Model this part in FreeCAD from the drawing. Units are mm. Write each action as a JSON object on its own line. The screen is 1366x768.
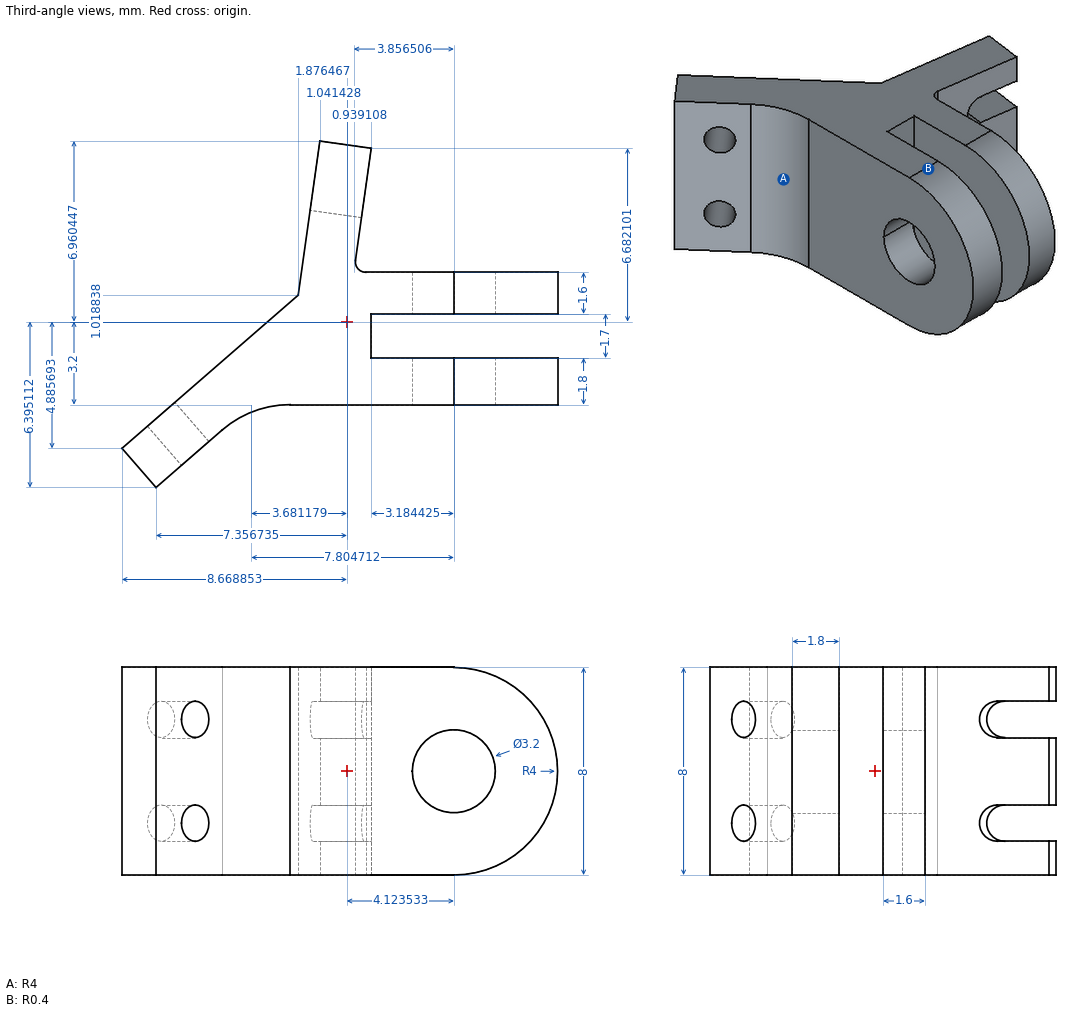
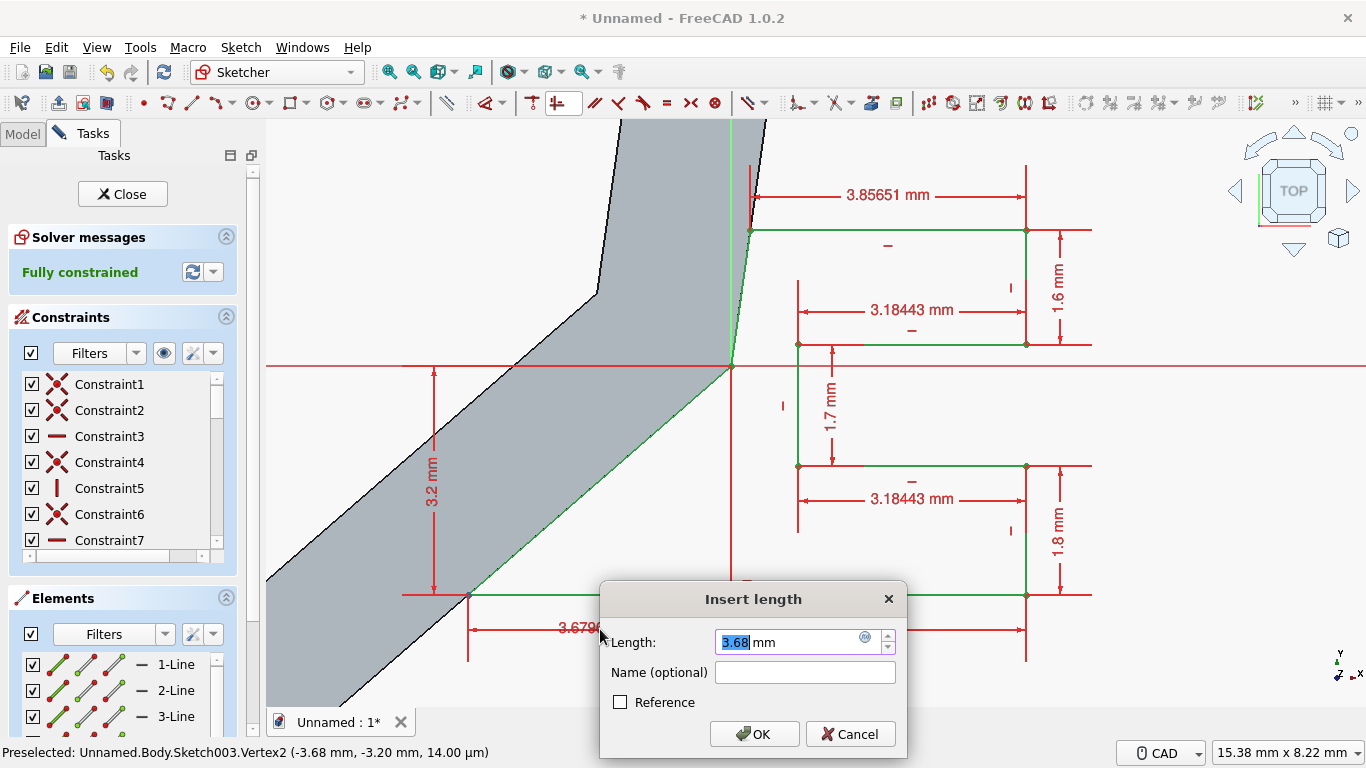
{"action": "type", "text": "3.681179"}
{"action": "key", "text": "Return"}
{"action": "key", "text": "Escape"}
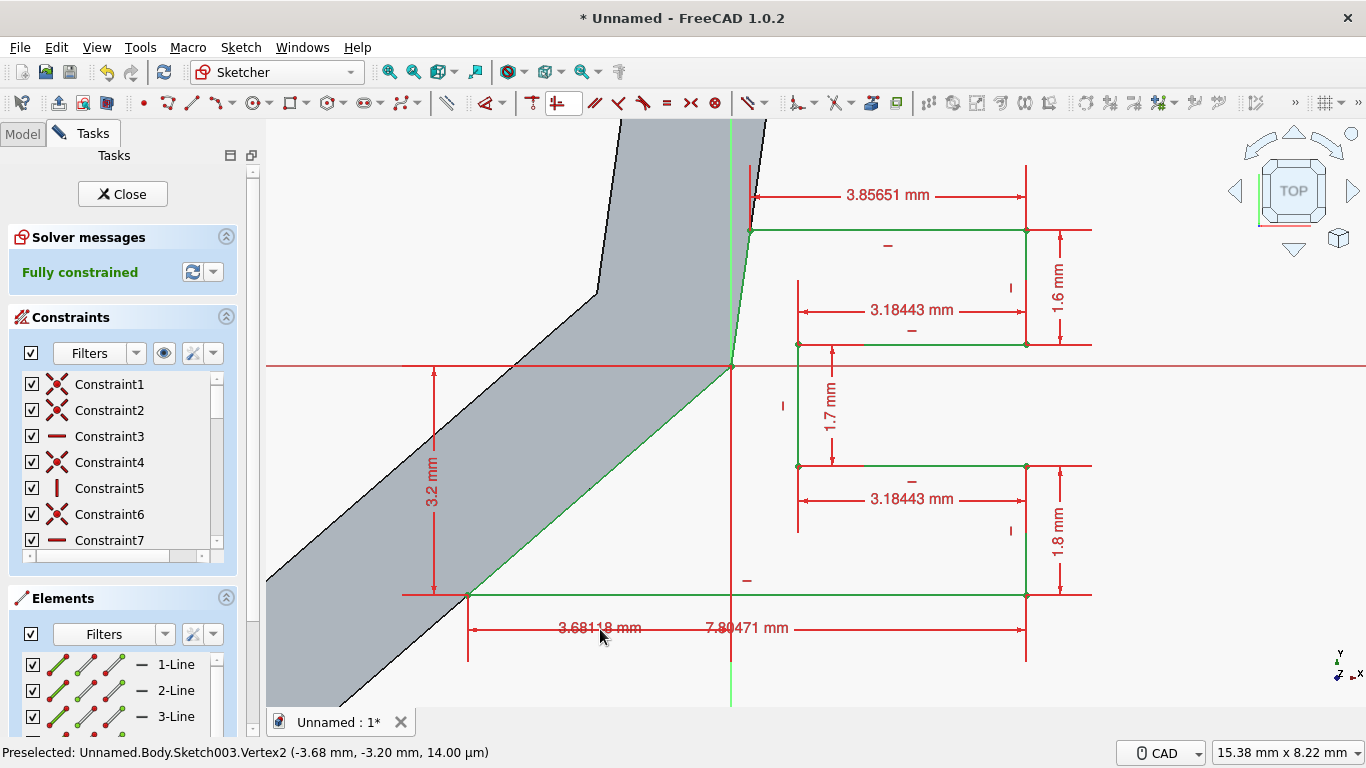
{"action": "left_click", "coordinate": [123, 194]}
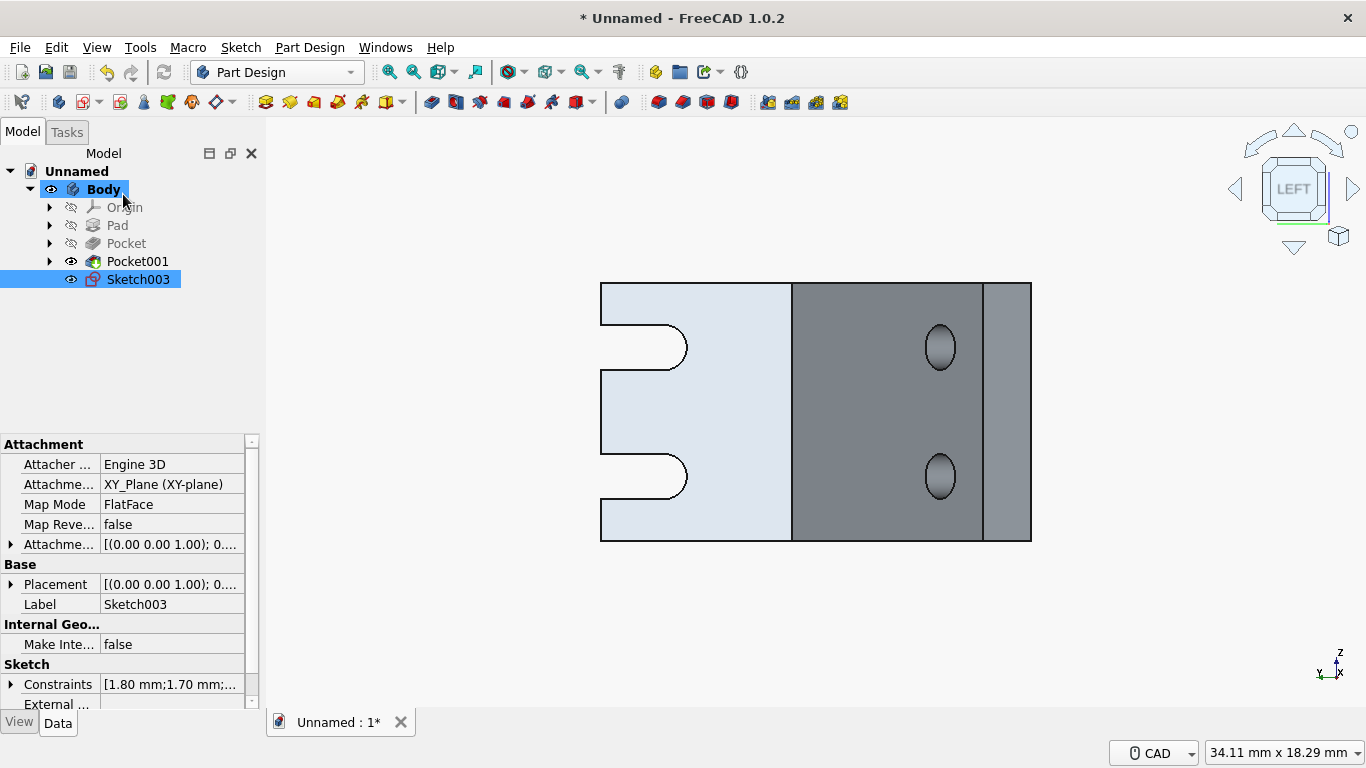
{"action": "left_click", "coordinate": [266, 102]}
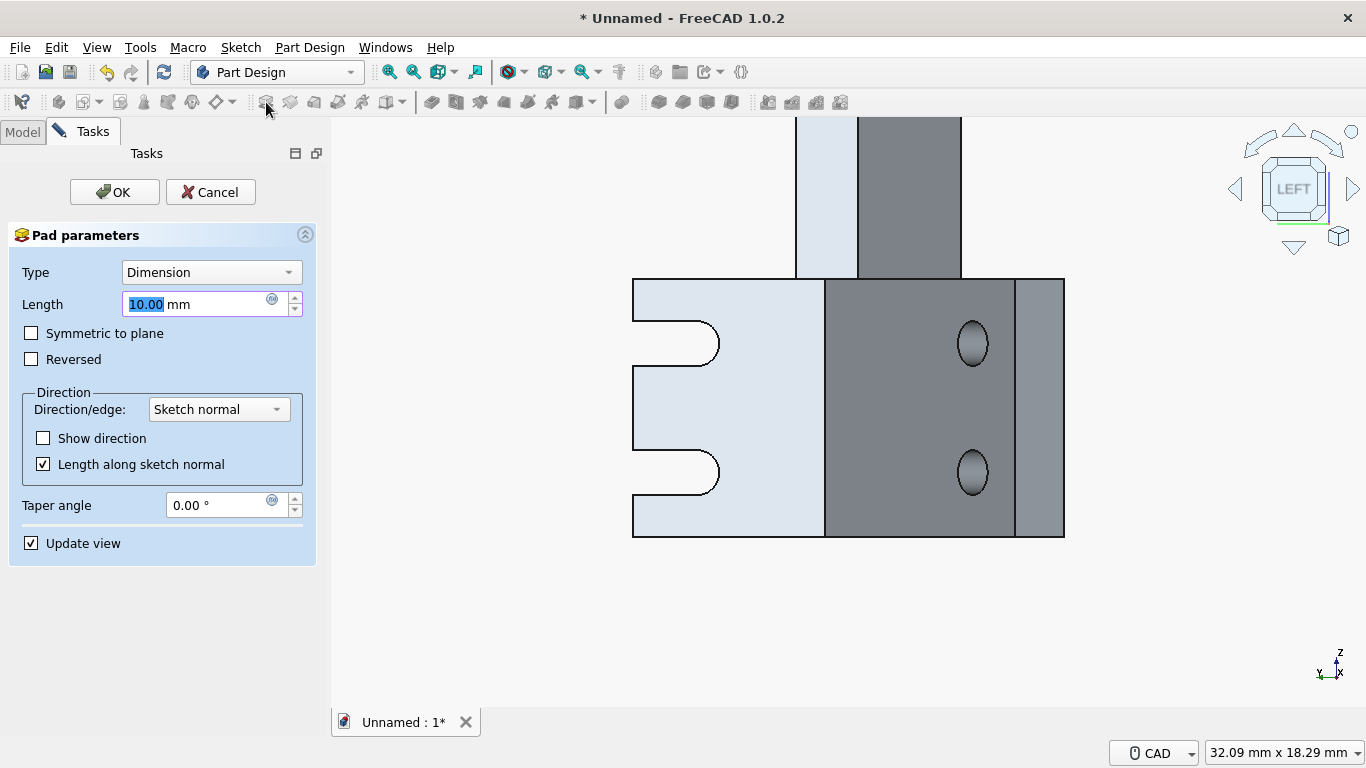
{"action": "type", "text": "8"}
{"action": "key", "text": "Tab"}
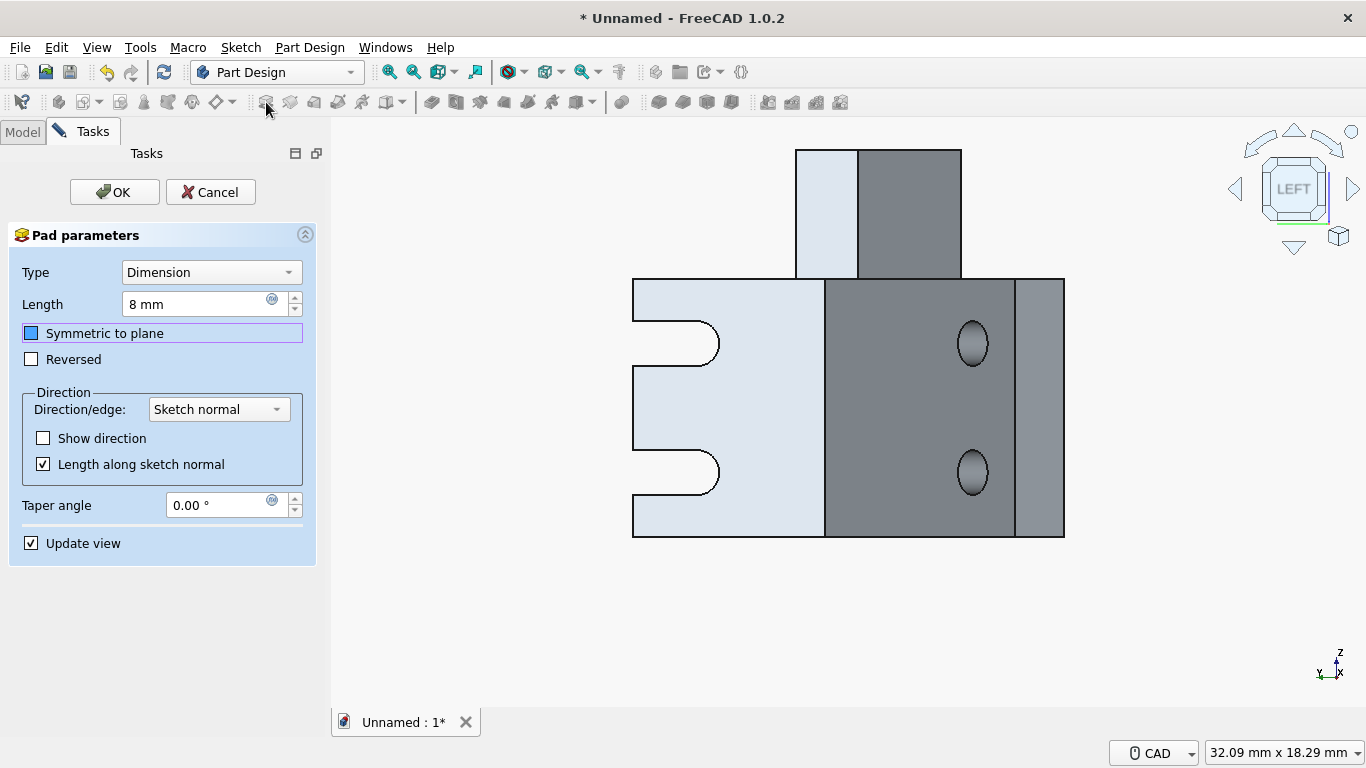
{"action": "left_click", "coordinate": [30, 333]}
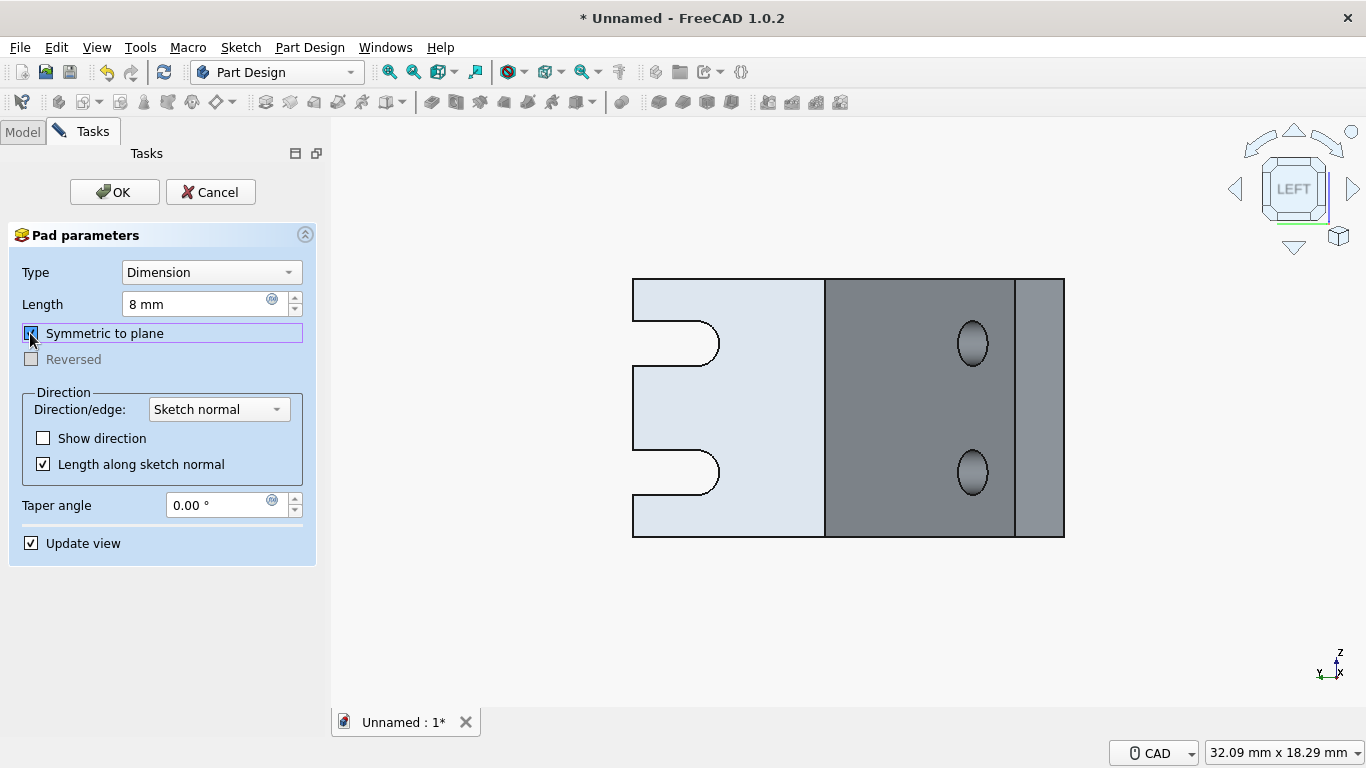
{"action": "left_click", "coordinate": [115, 192]}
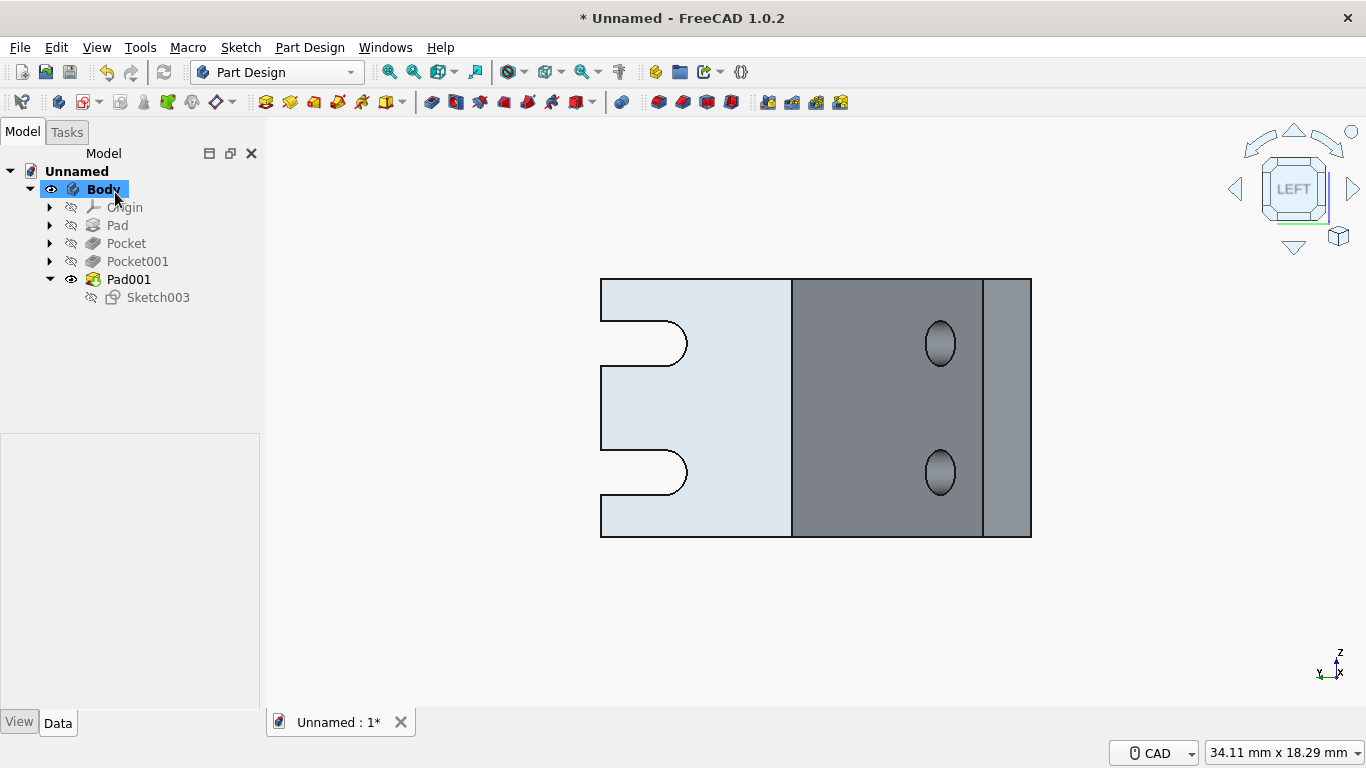
{"action": "left_click", "coordinate": [390, 72]}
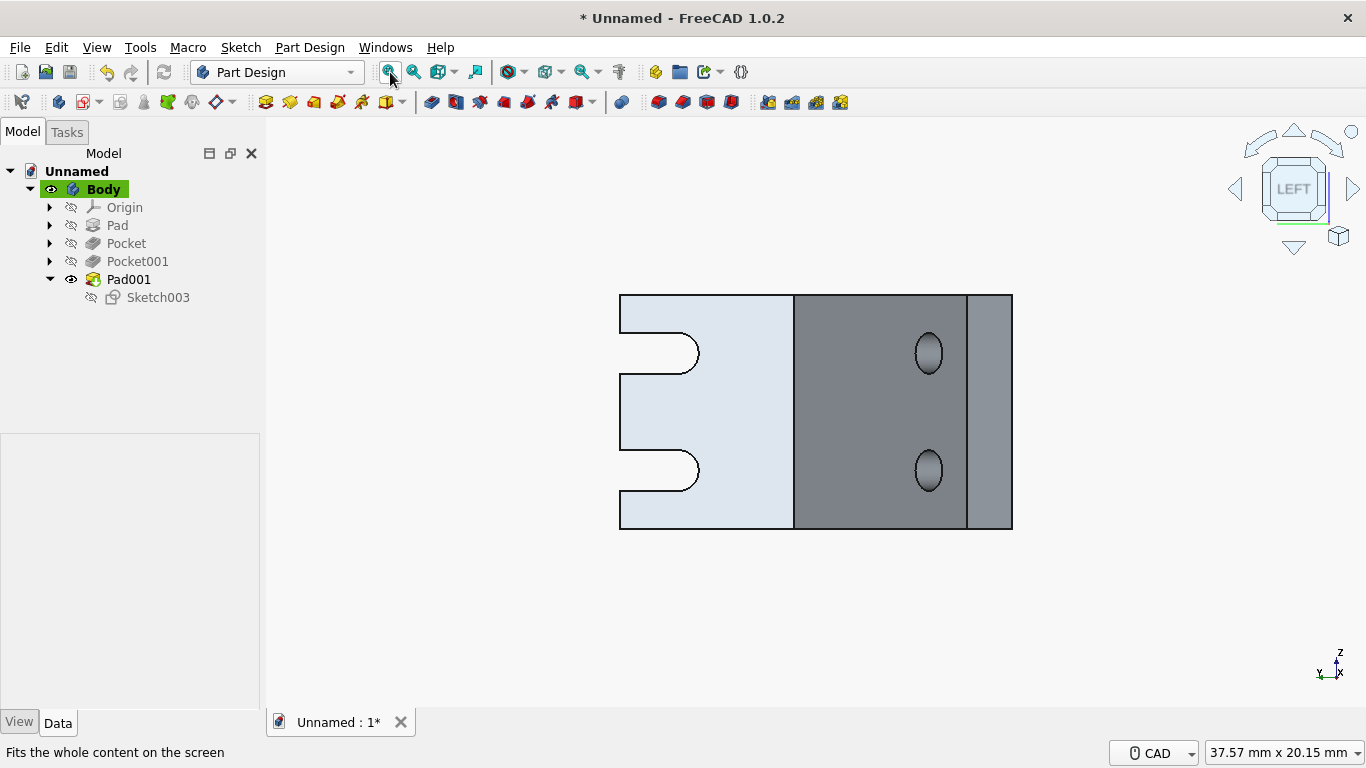
{"action": "key", "text": "0"}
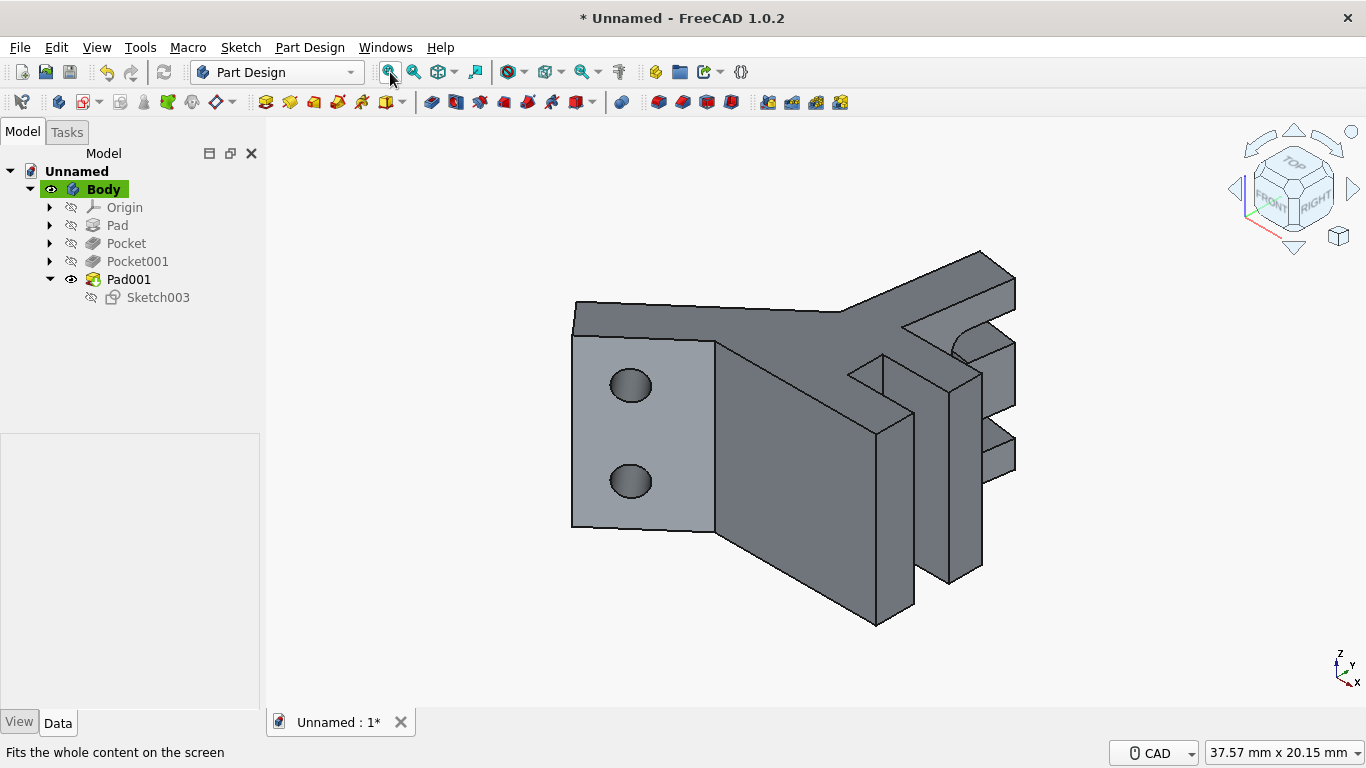
{"action": "key", "text": "2"}